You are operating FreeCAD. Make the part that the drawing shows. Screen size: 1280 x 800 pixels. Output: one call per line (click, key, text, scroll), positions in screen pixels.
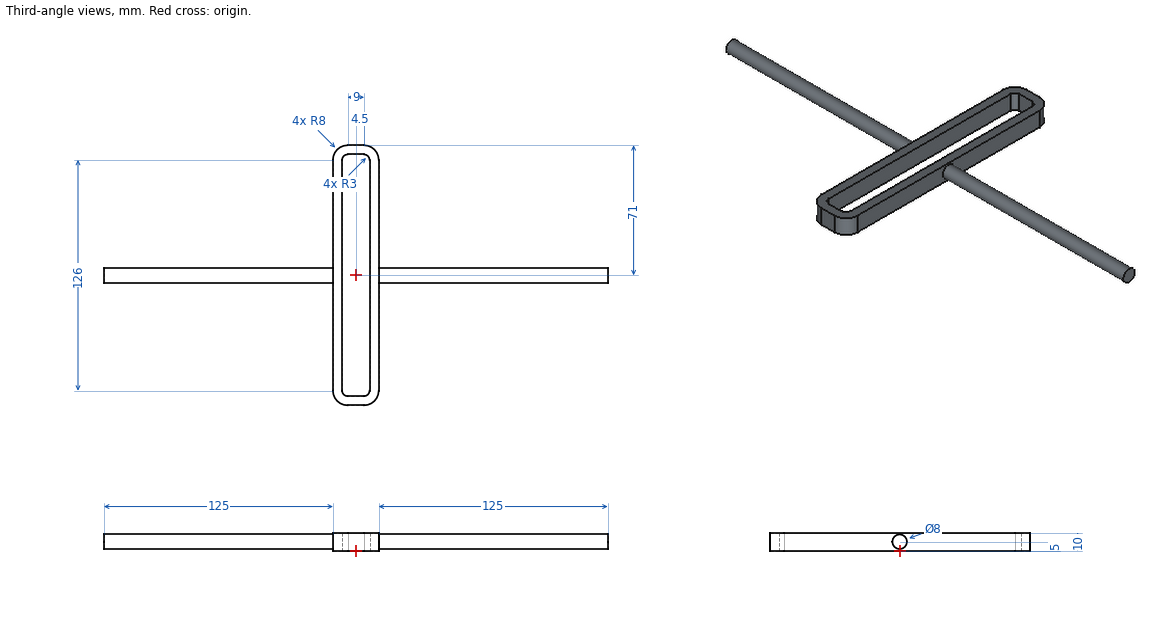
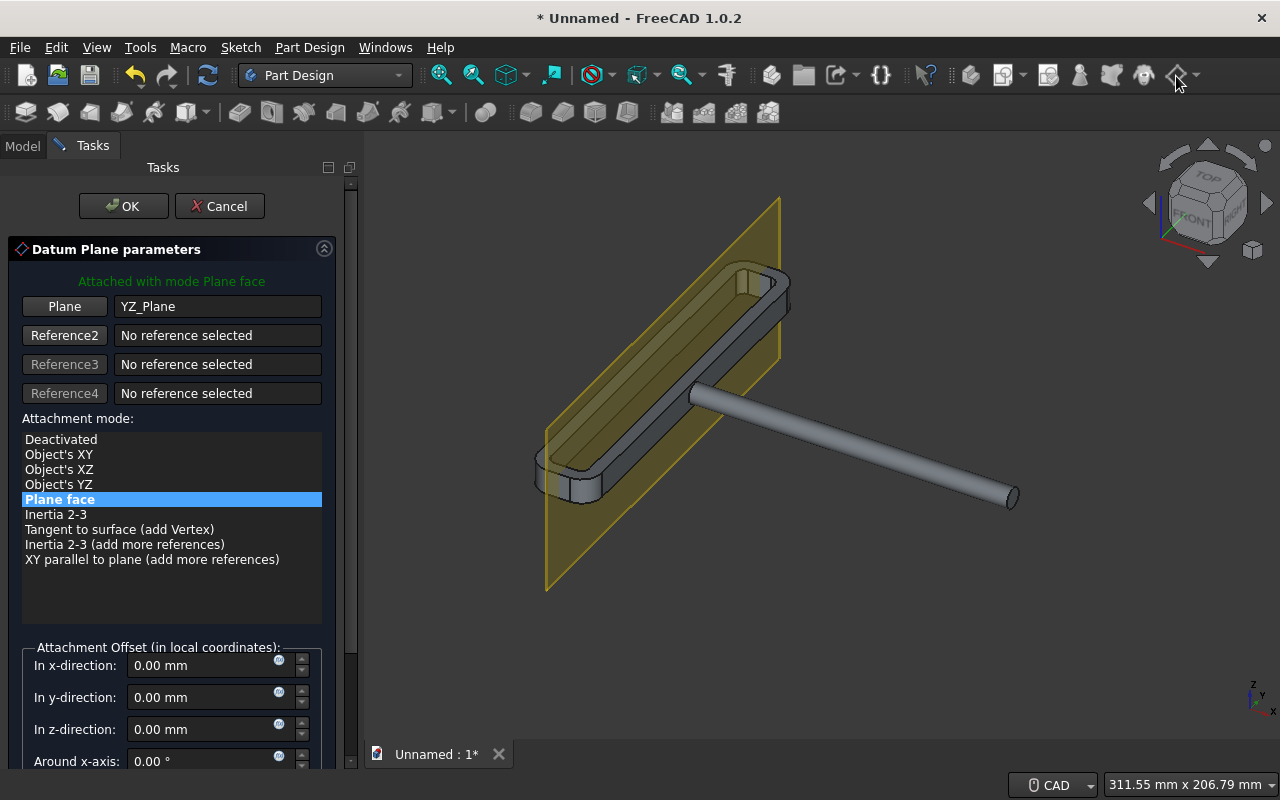
triple_click(210, 729)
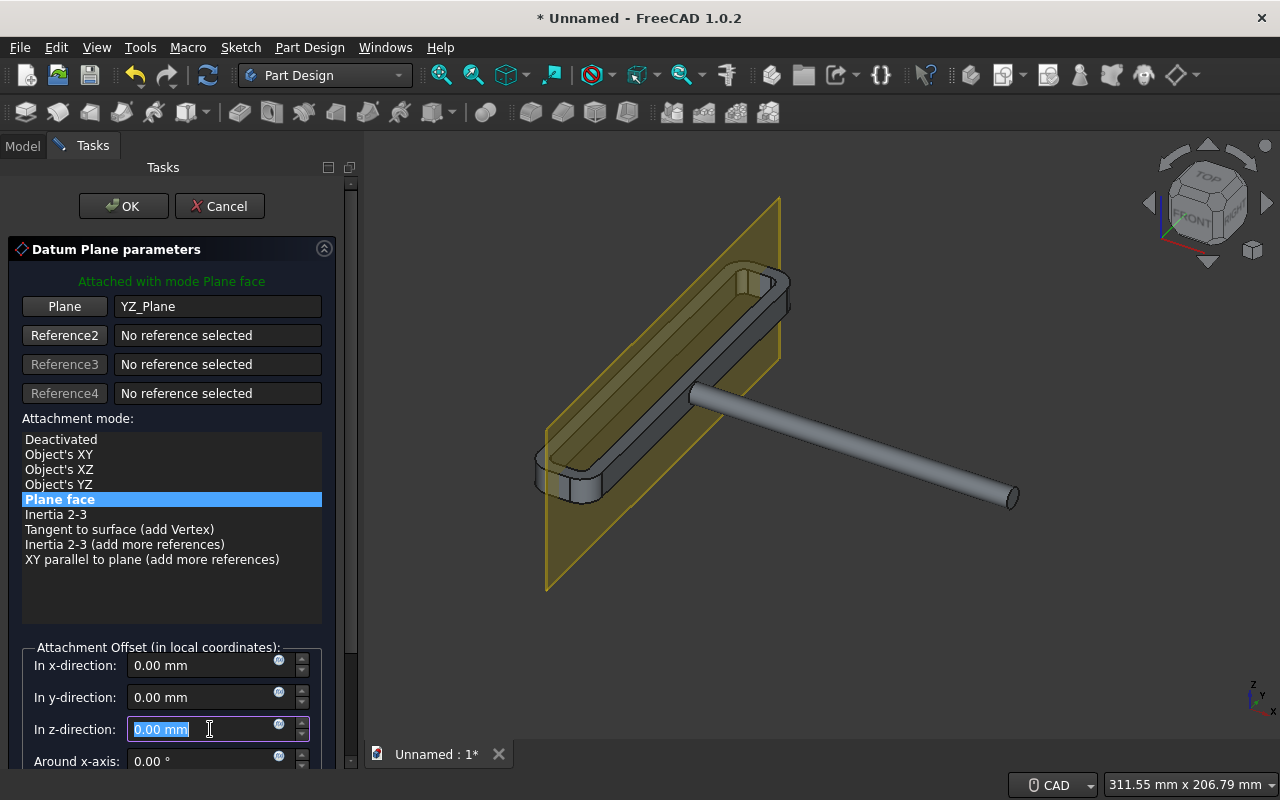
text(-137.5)
key(Tab)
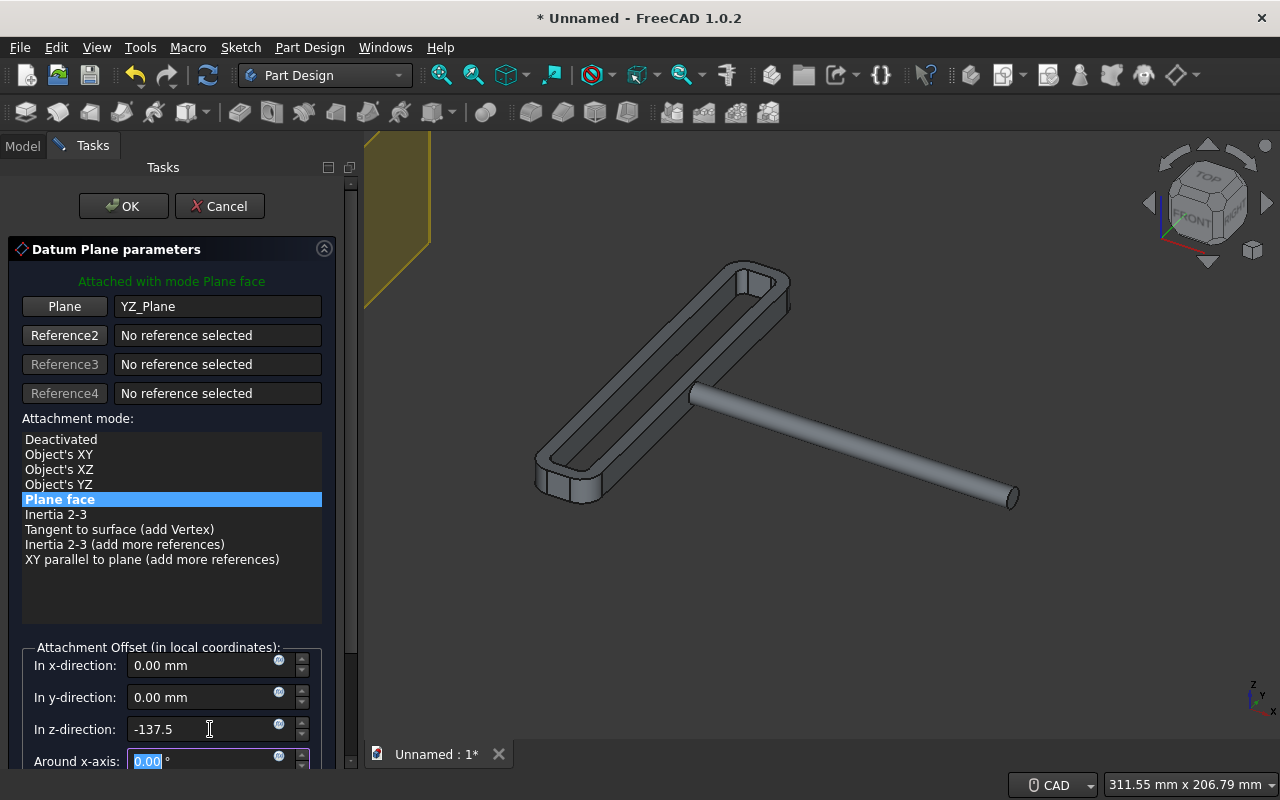
click(124, 206)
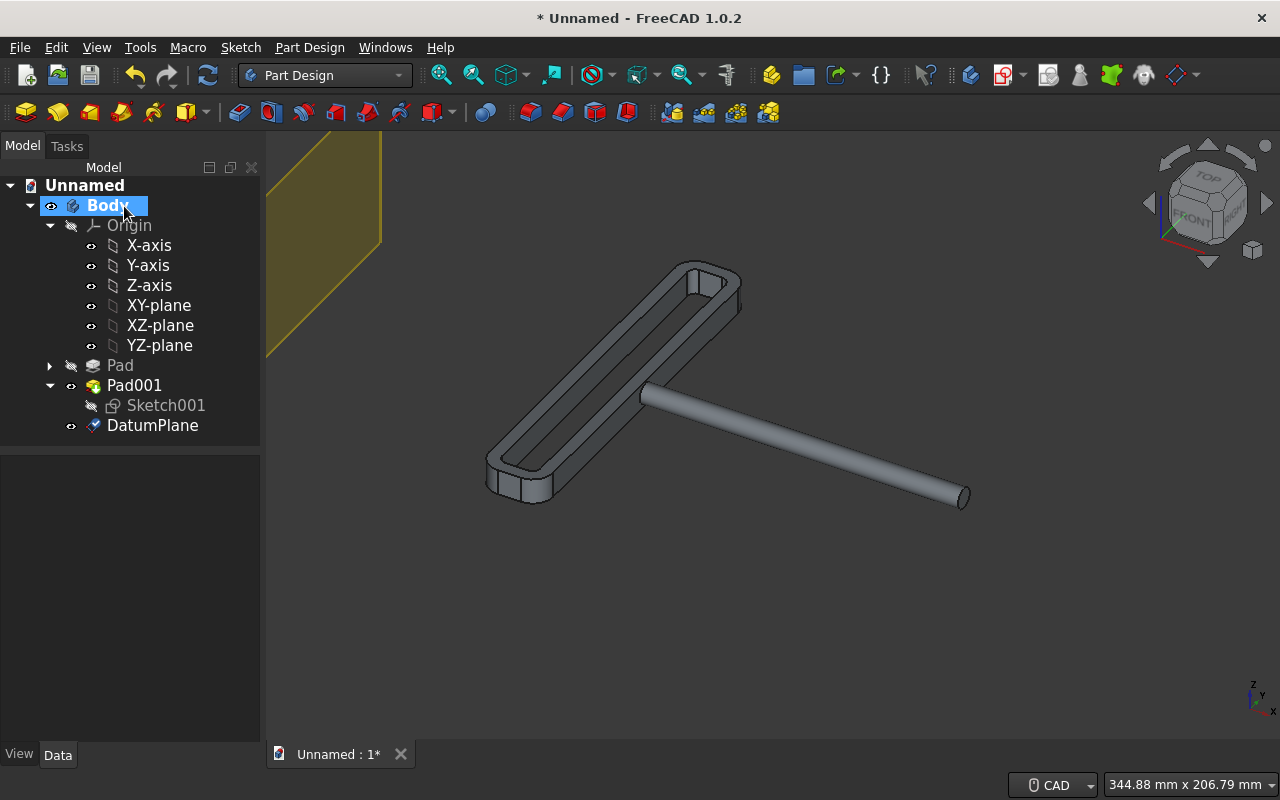
click(116, 426)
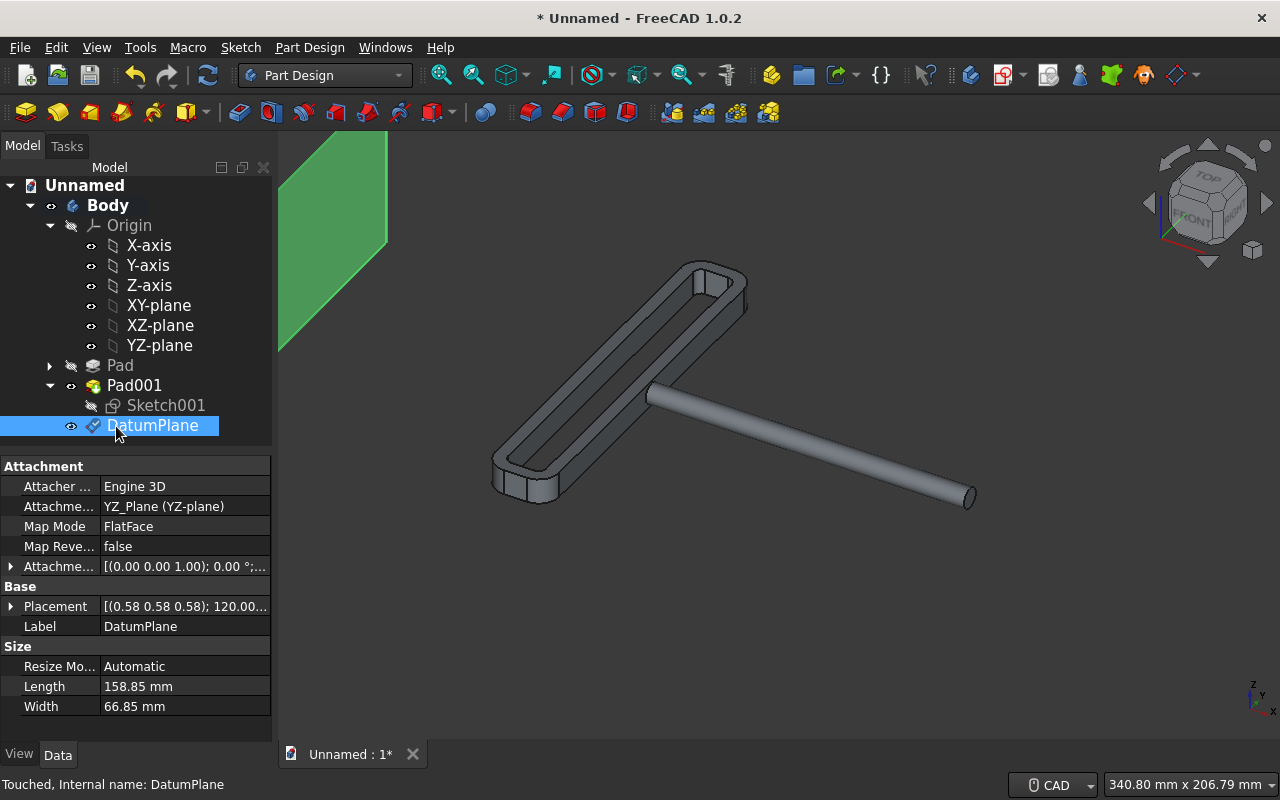
click(1004, 76)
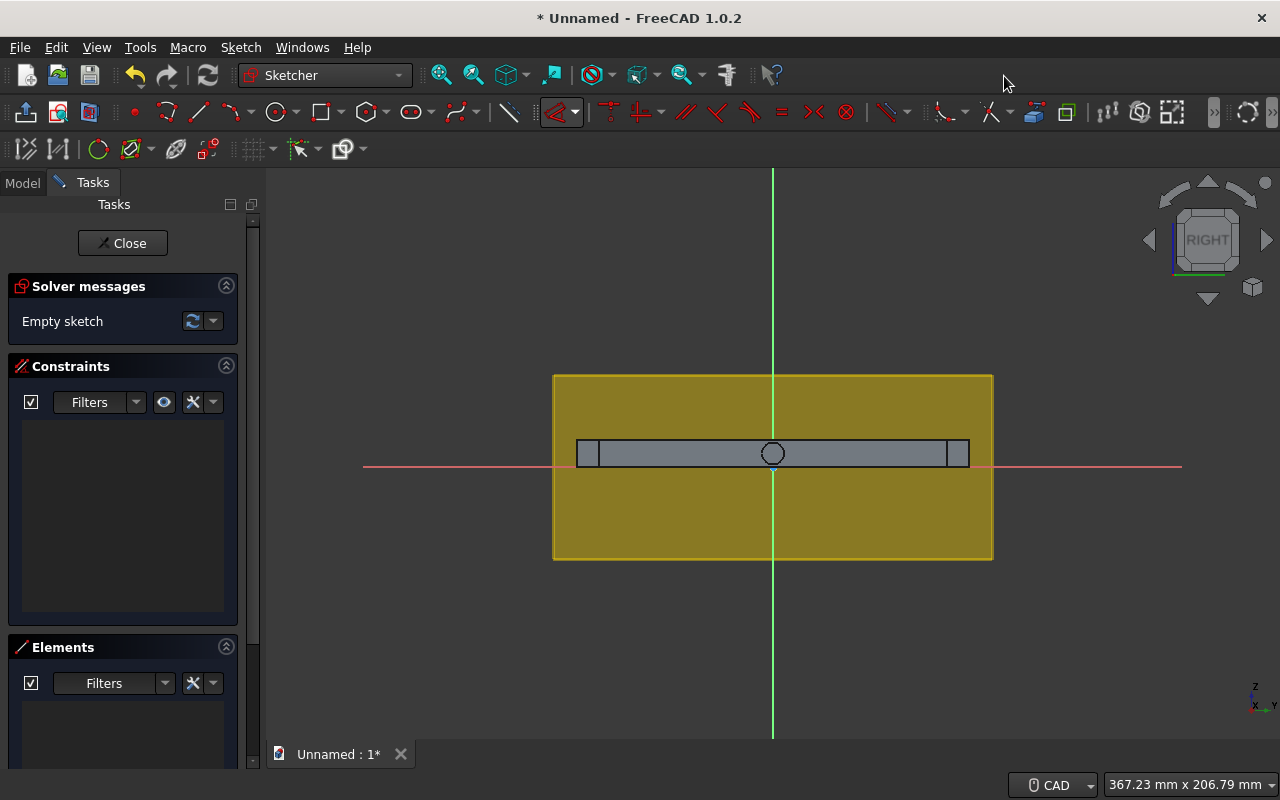
click(90, 112)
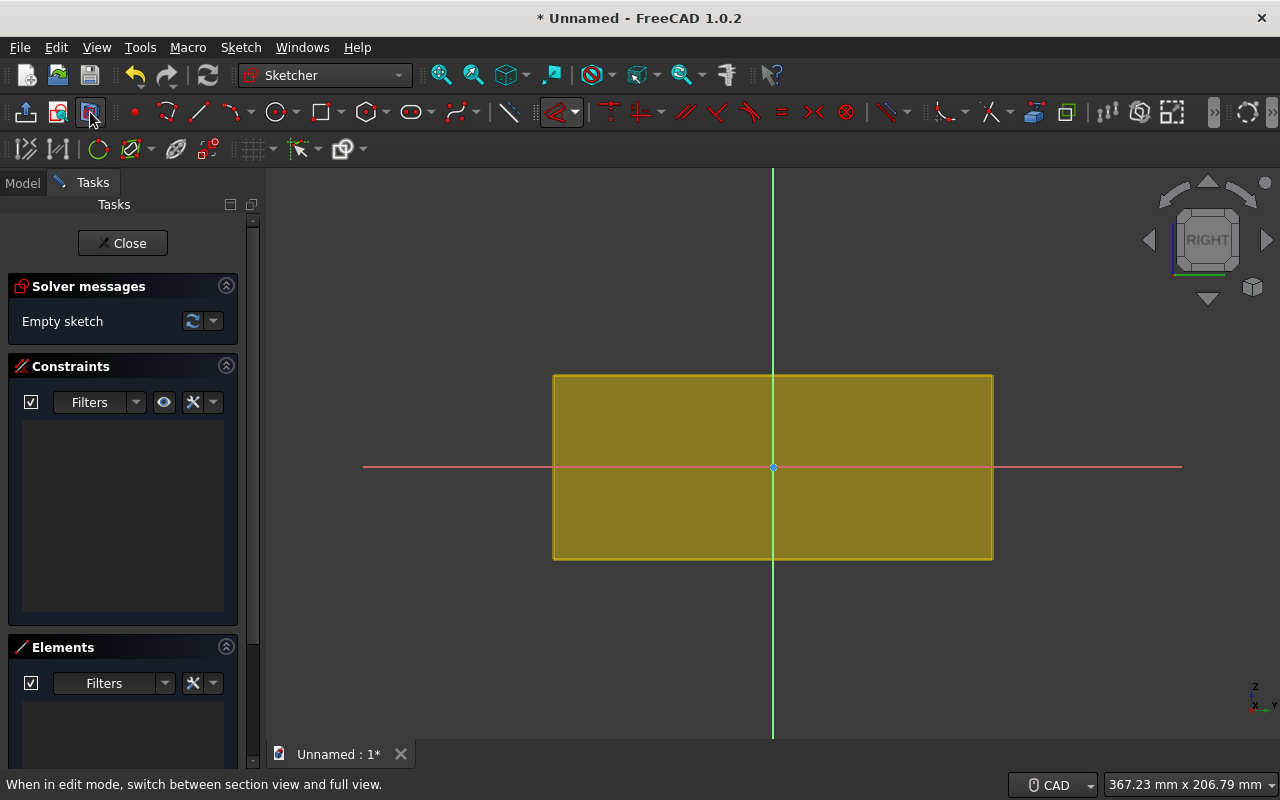
scroll(778, 455, up, 13)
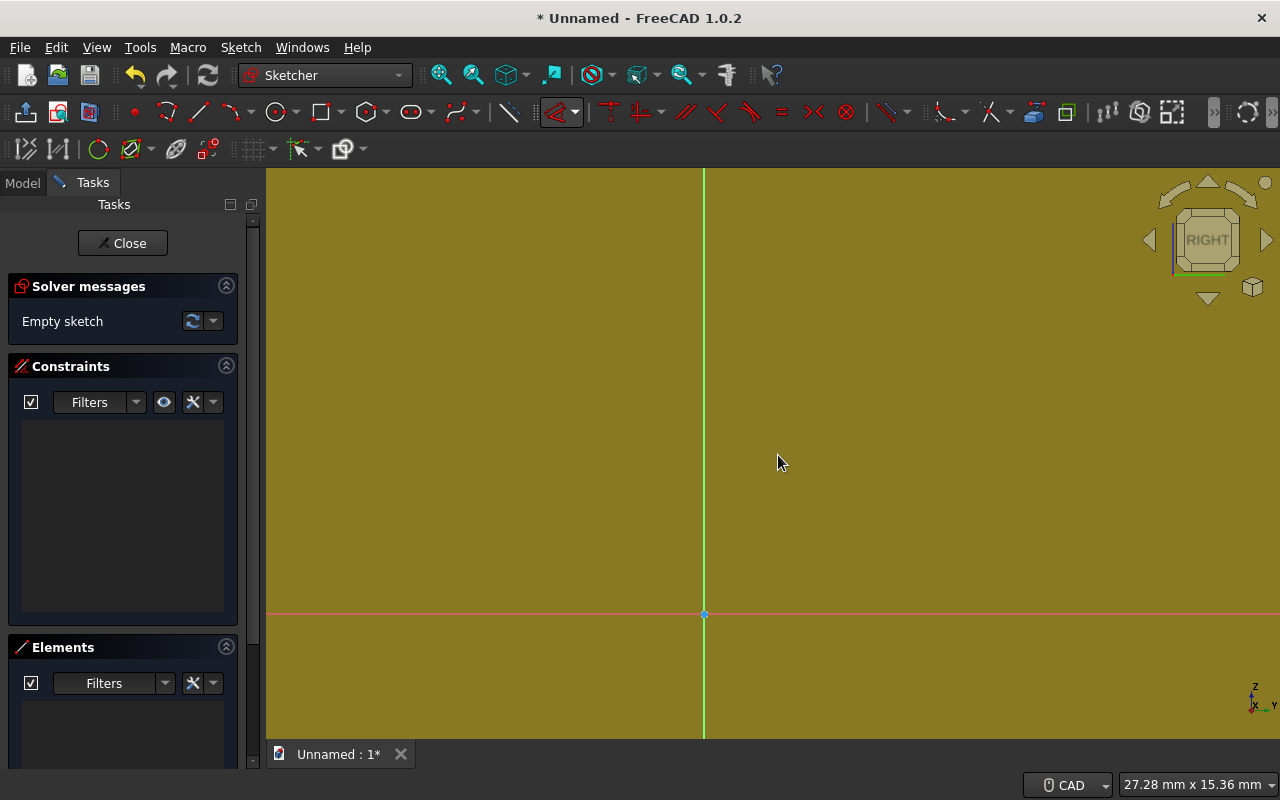
click(276, 112)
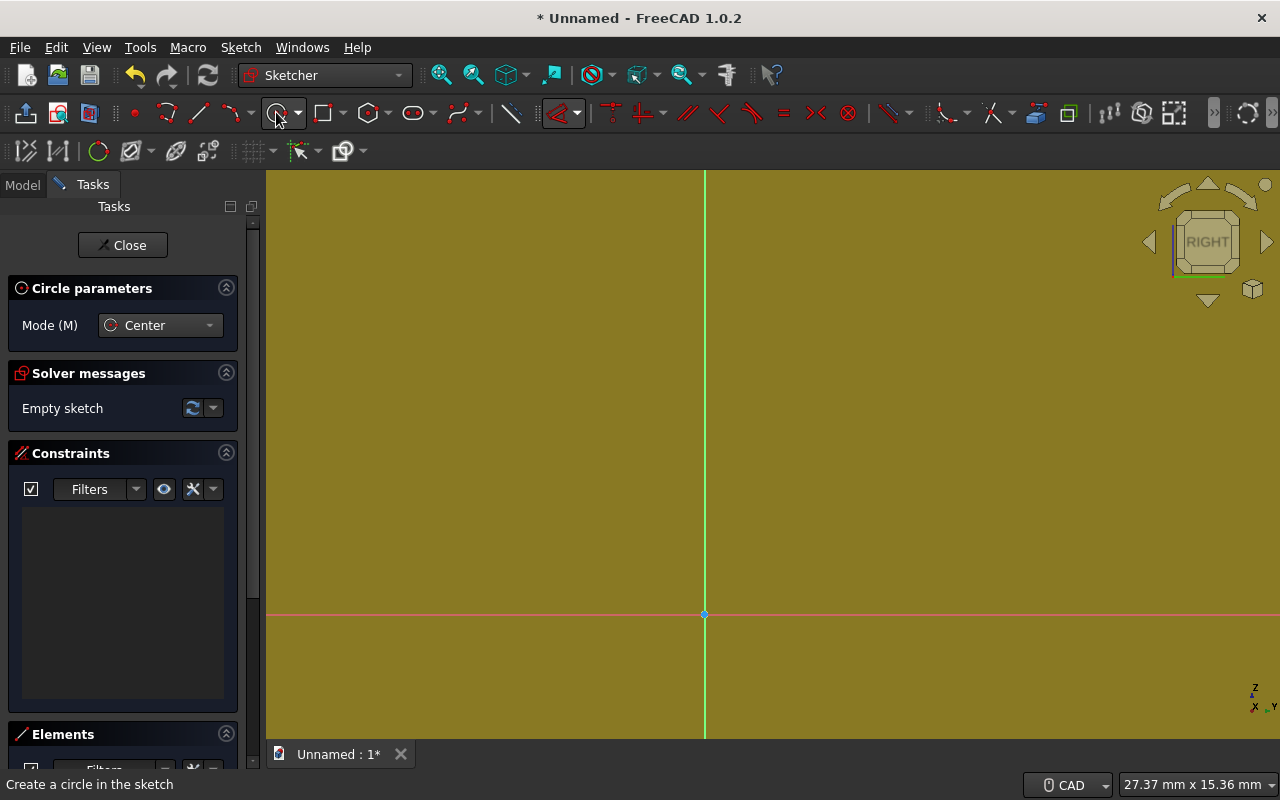
click(705, 430)
click(809, 325)
key(Escape)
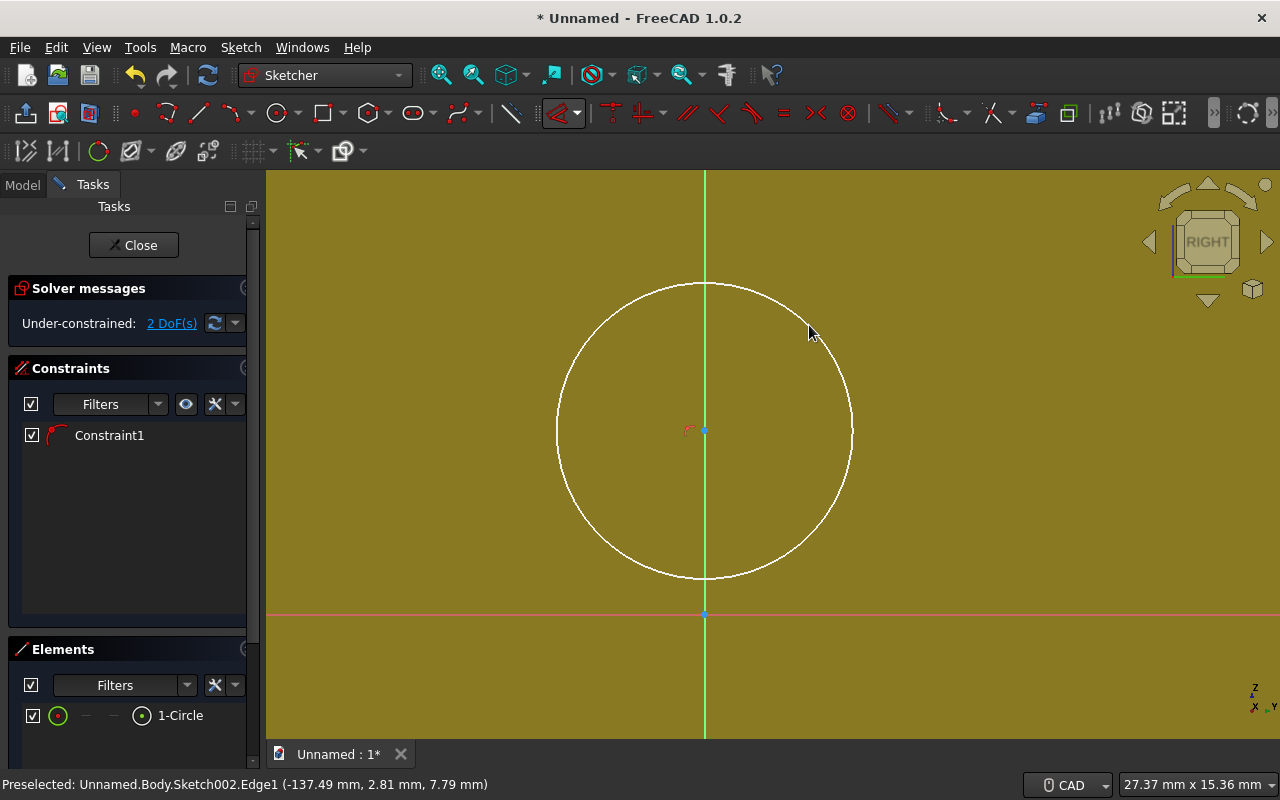
click(809, 326)